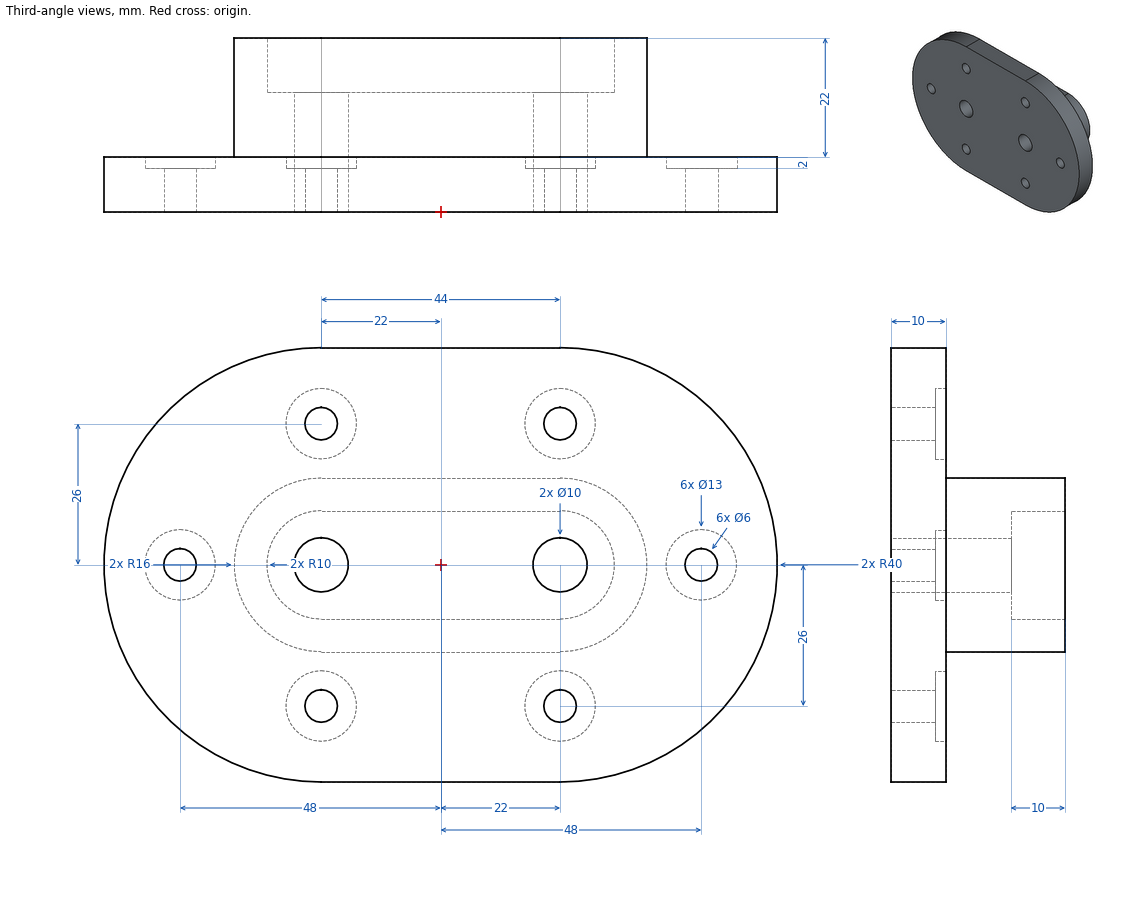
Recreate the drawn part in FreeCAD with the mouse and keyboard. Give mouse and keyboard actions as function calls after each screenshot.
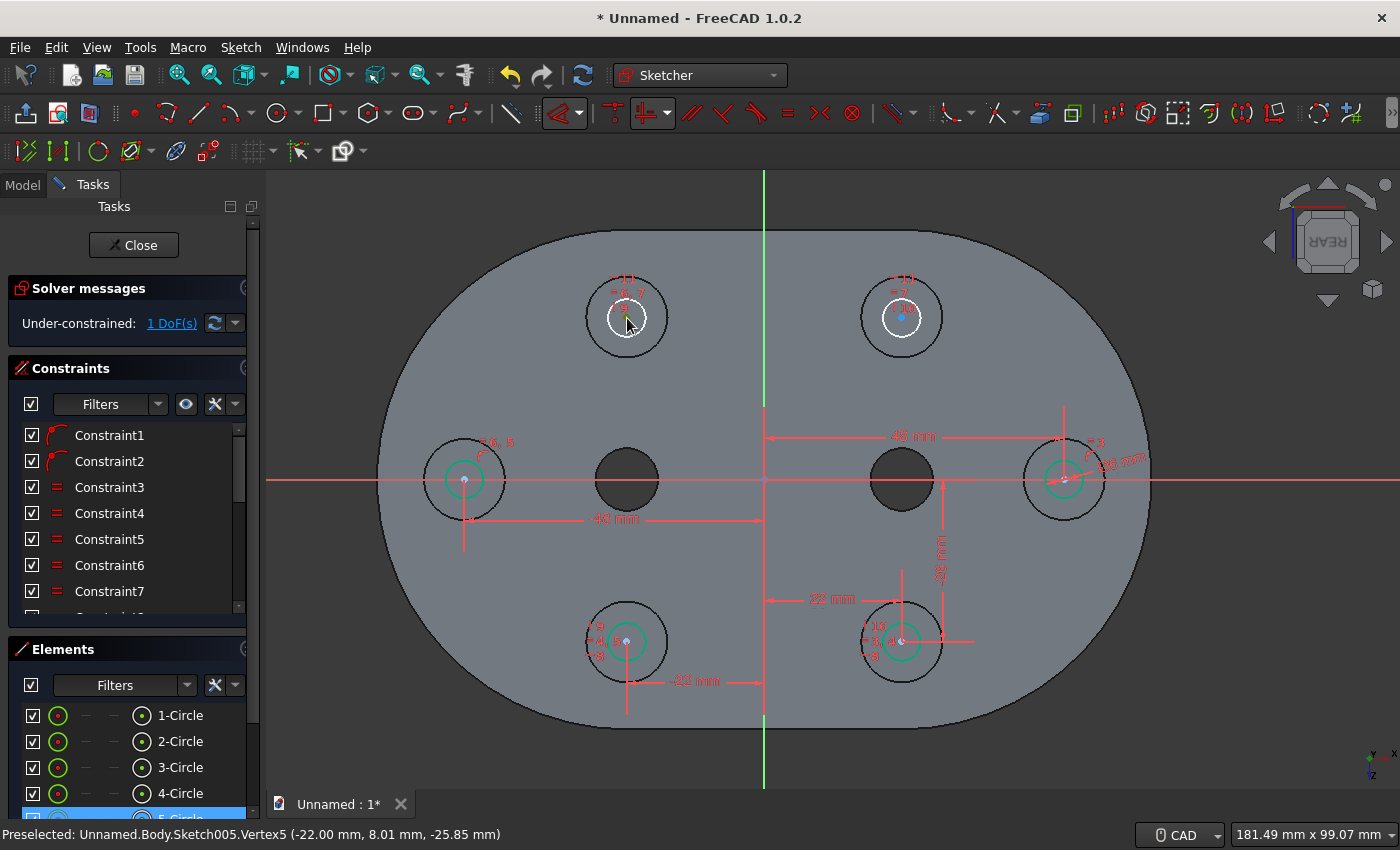
click(582, 114)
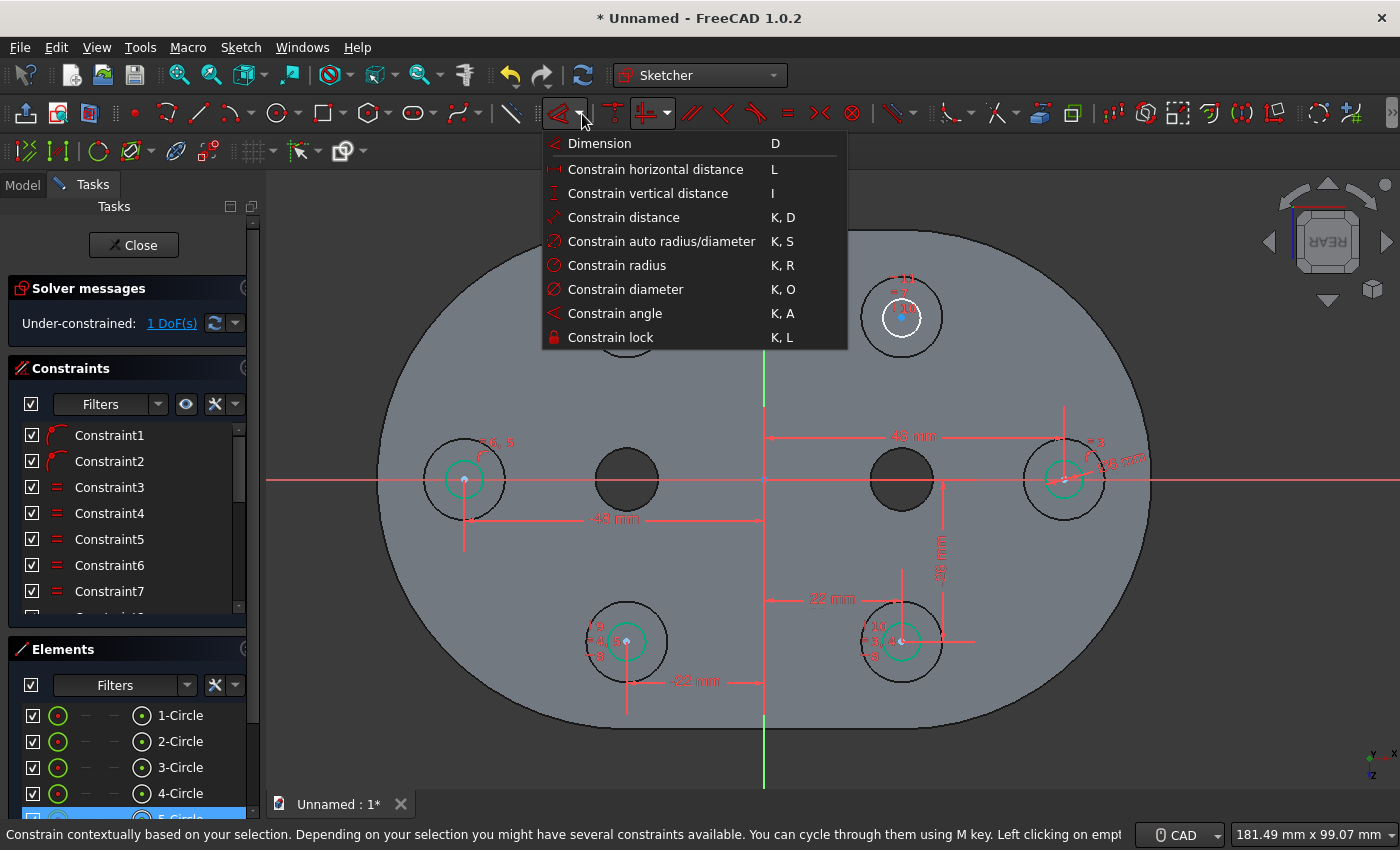
click(695, 193)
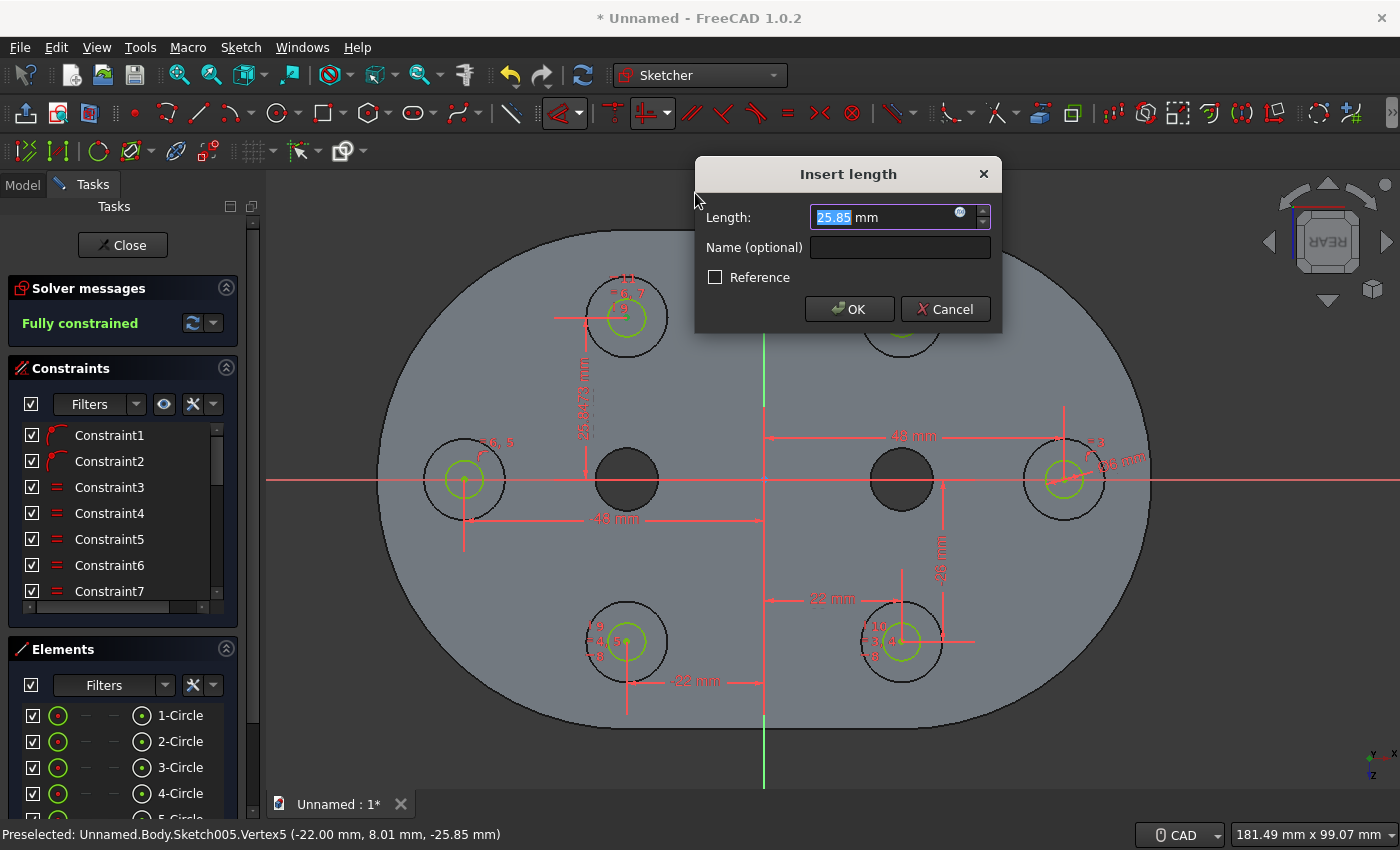
text(26)
key(Return)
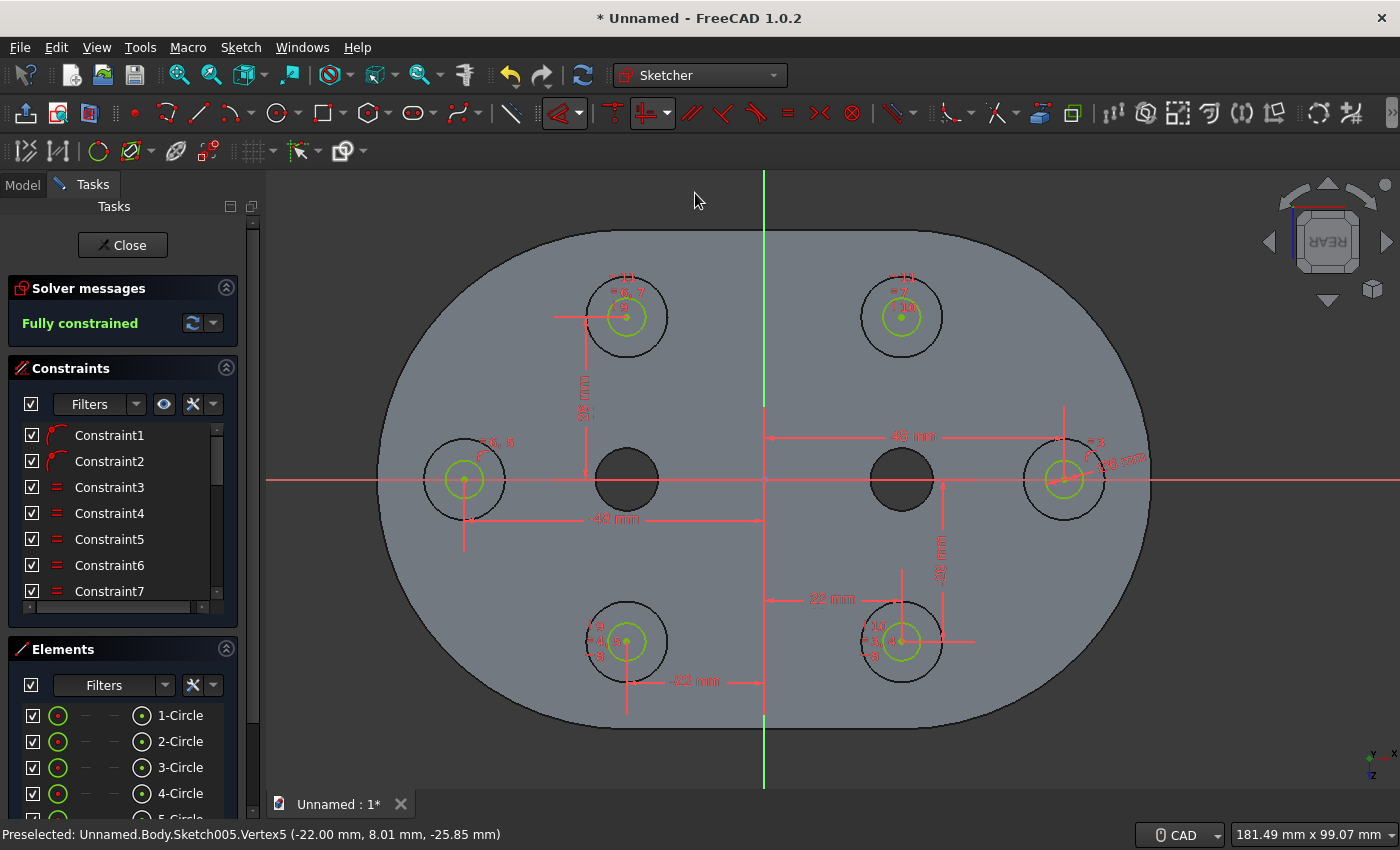
click(123, 245)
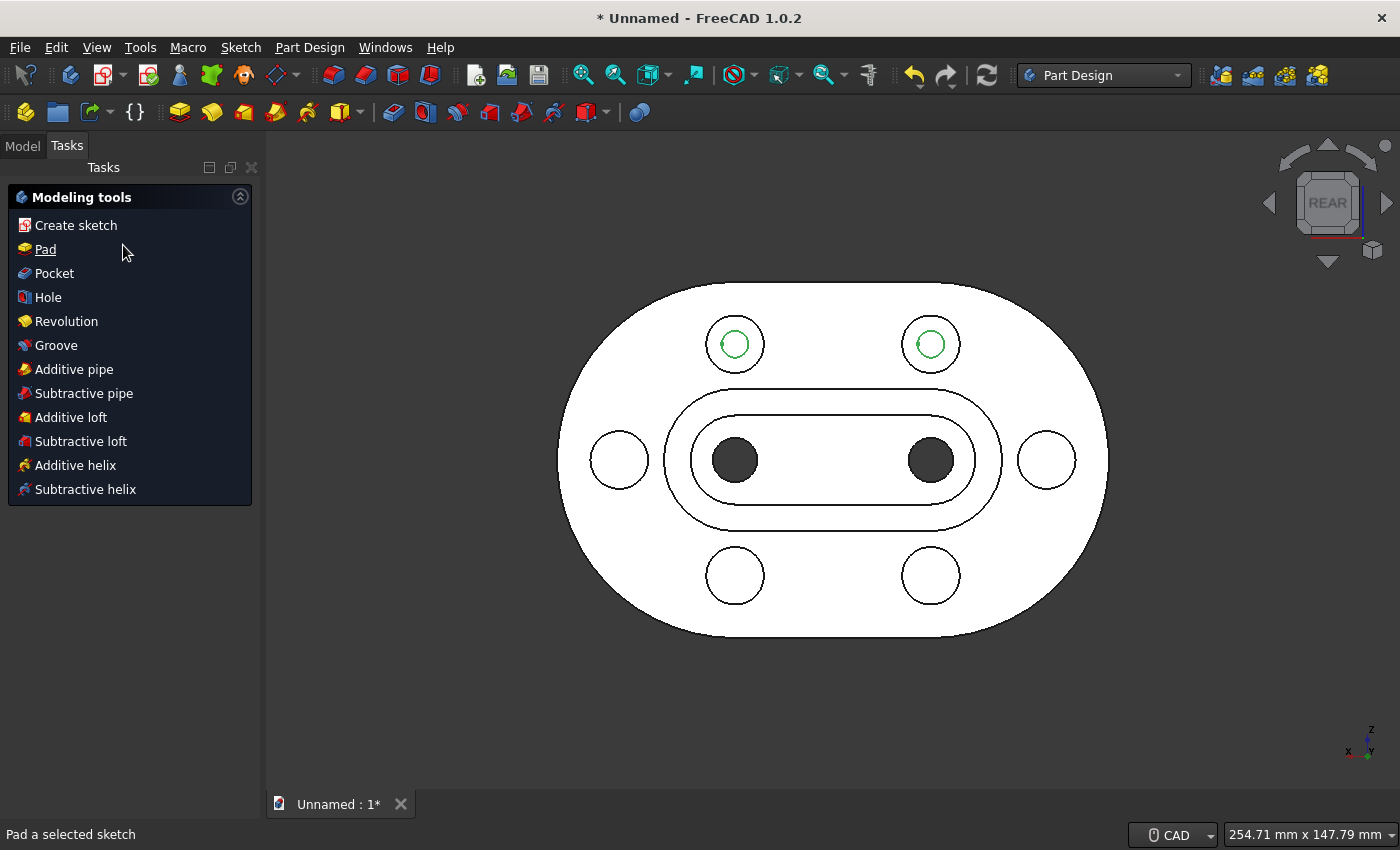
click(394, 112)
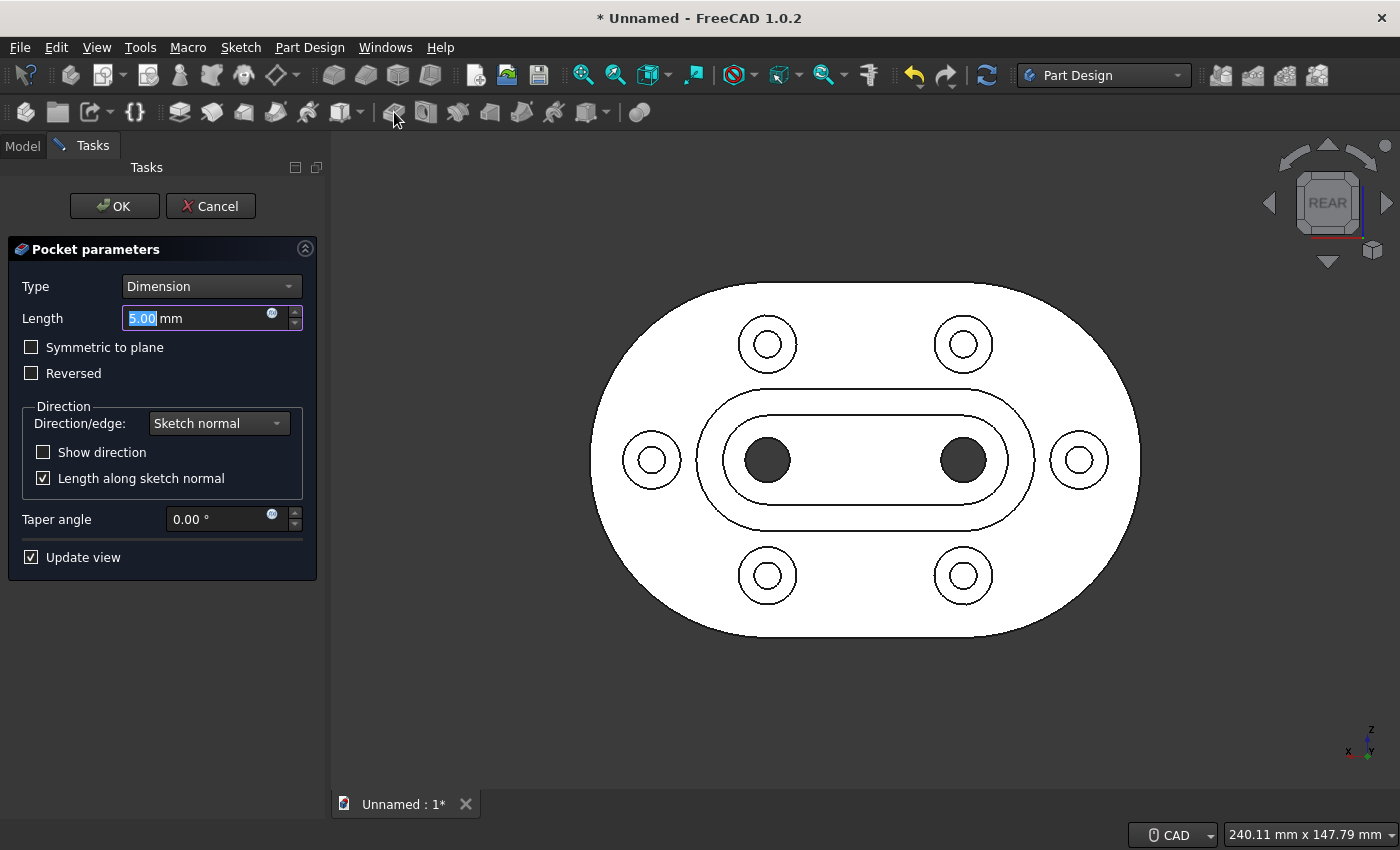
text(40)
key(Tab)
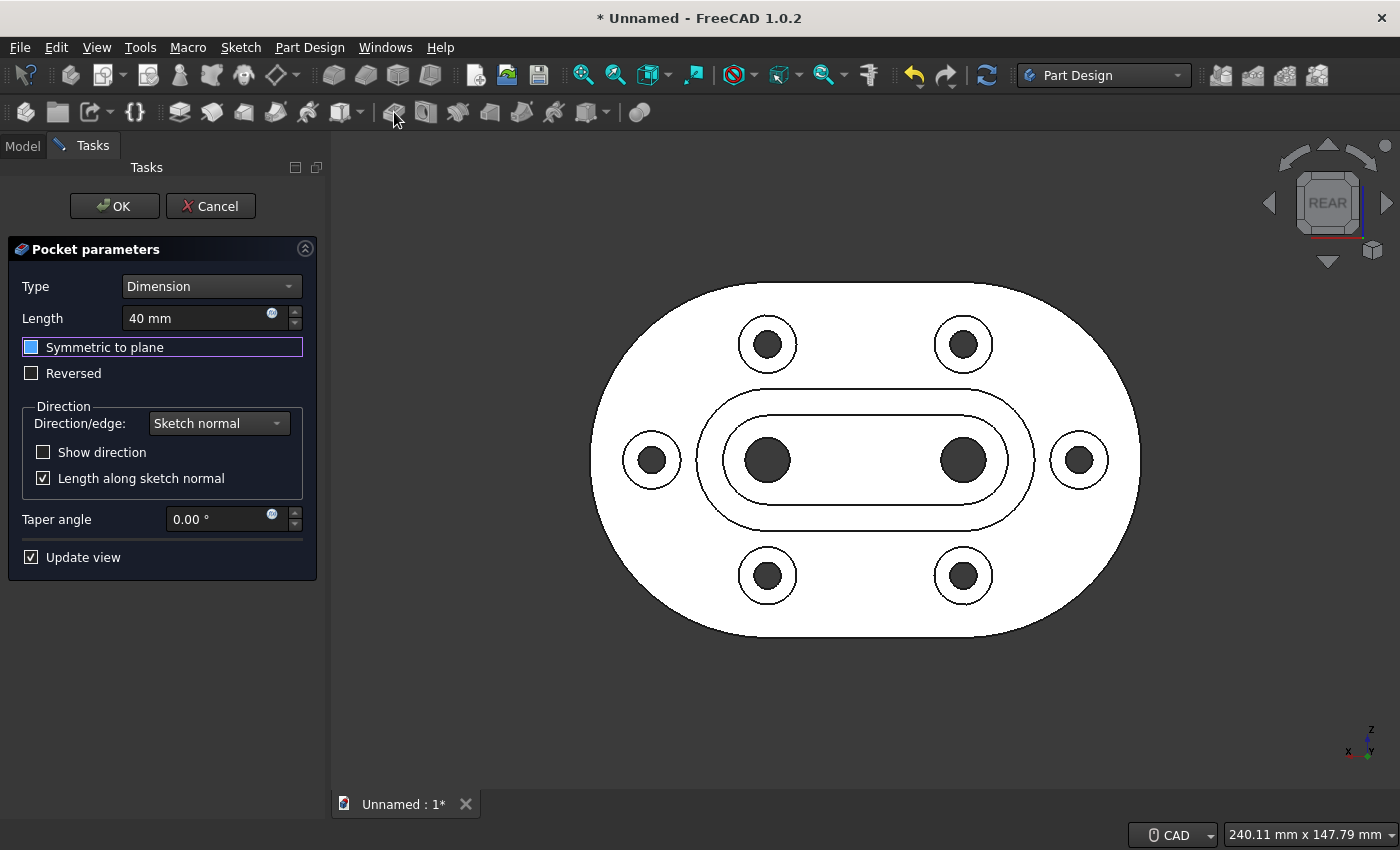
click(115, 206)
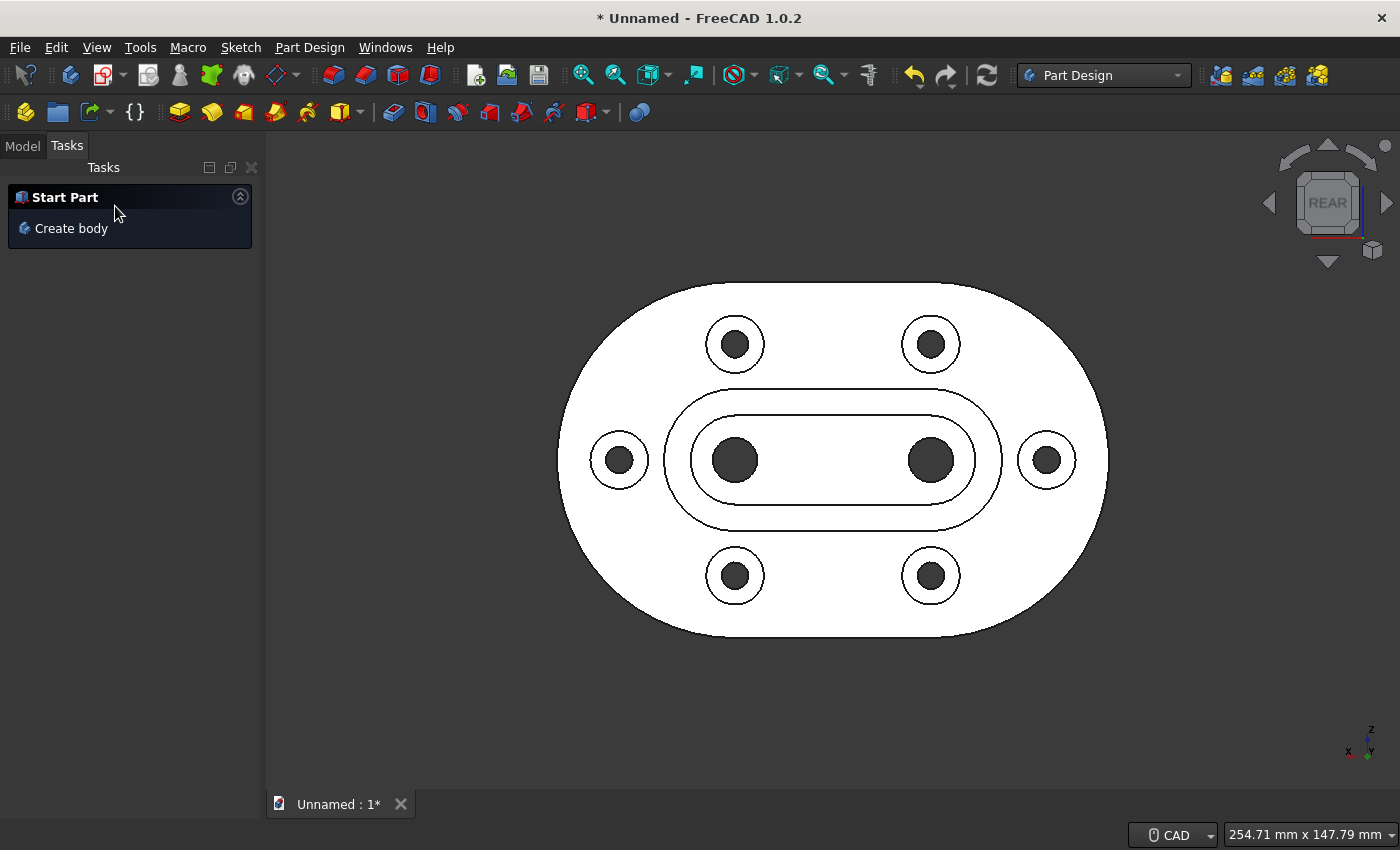
key(0)